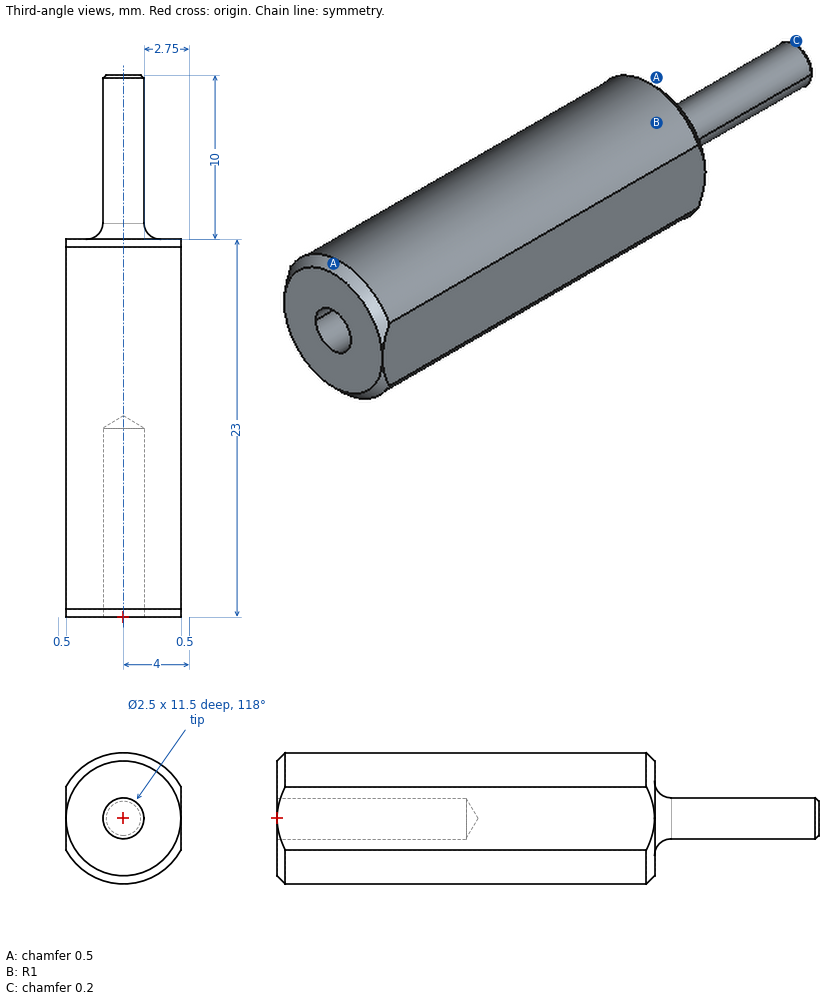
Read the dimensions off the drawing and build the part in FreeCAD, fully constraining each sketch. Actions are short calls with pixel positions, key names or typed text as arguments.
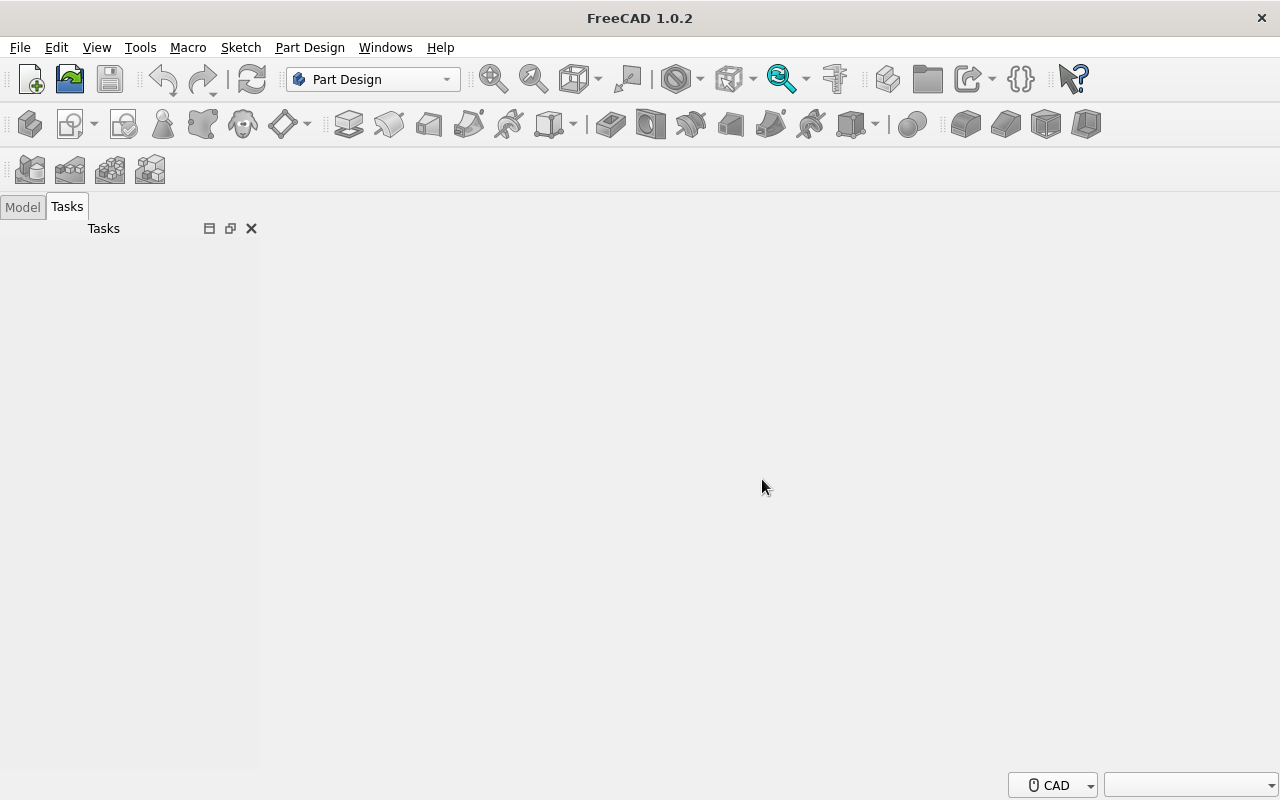
click(30, 80)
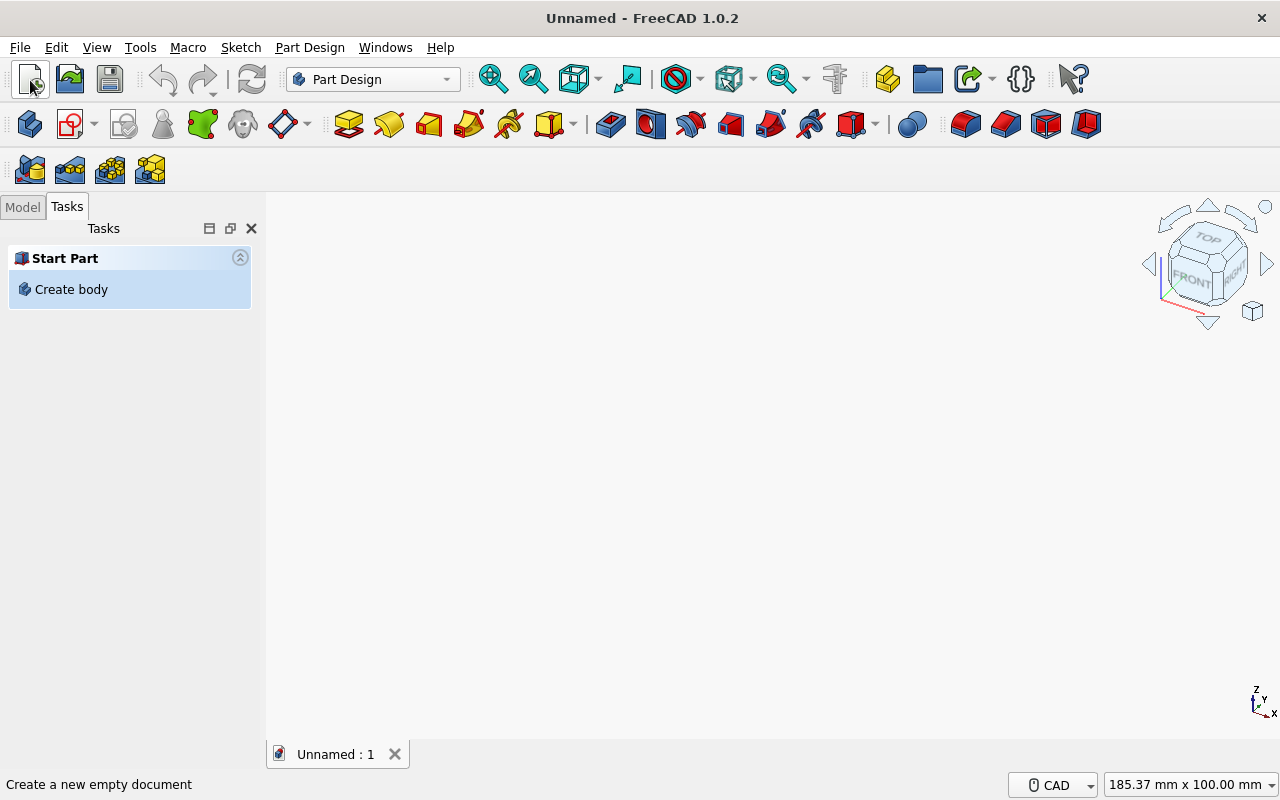
click(70, 124)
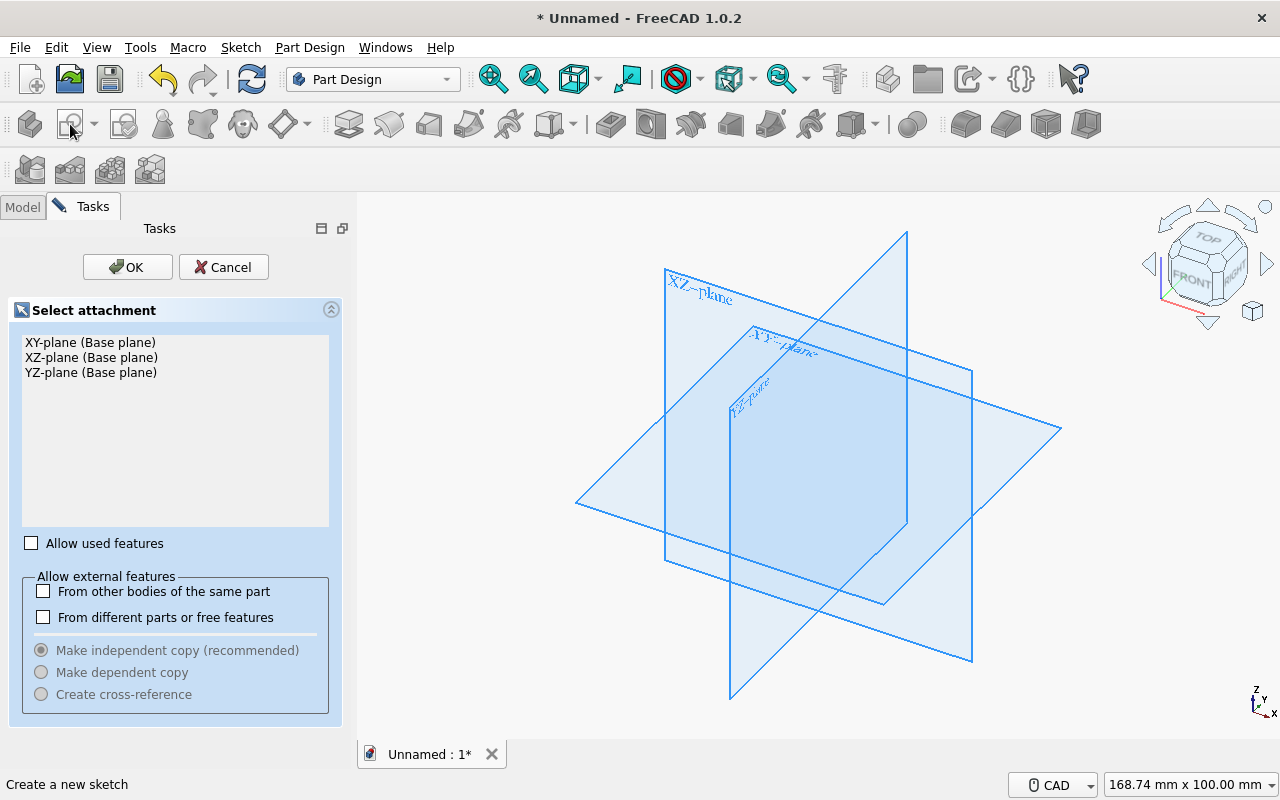
click(82, 342)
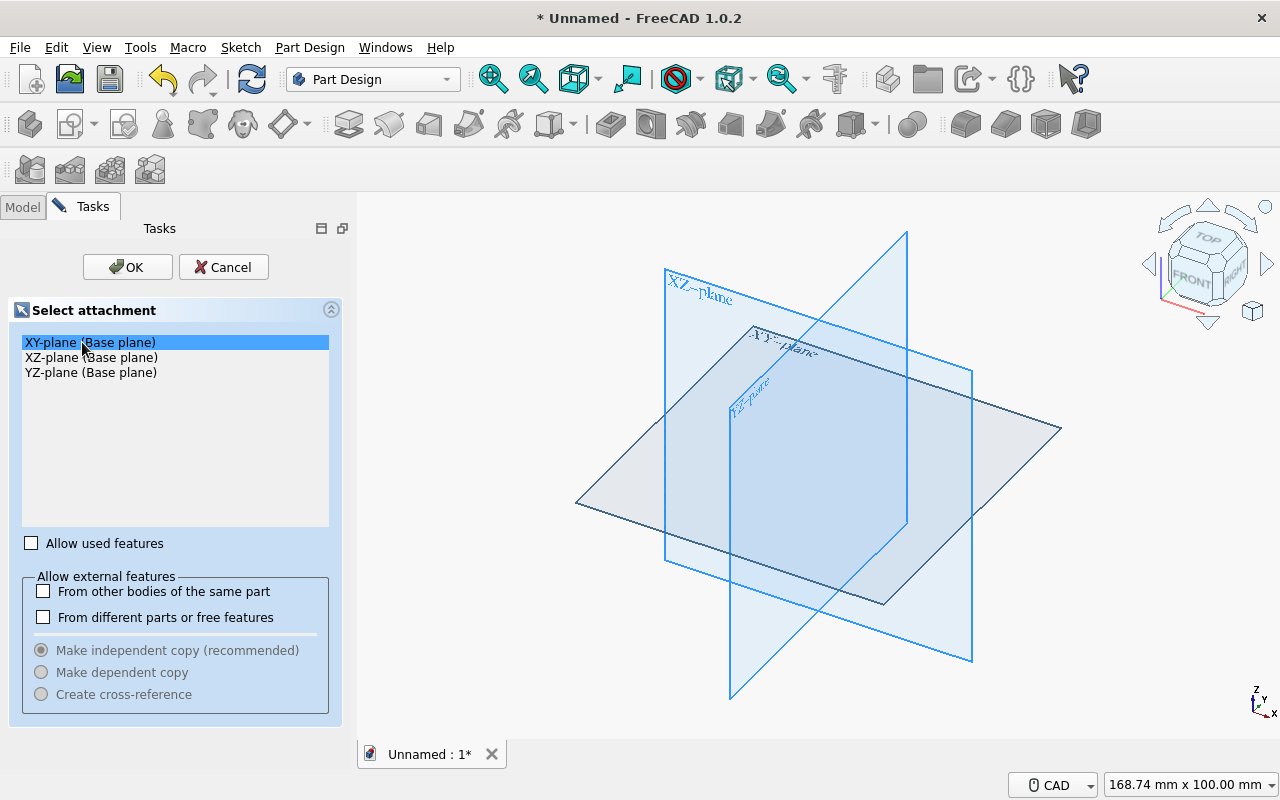
click(128, 267)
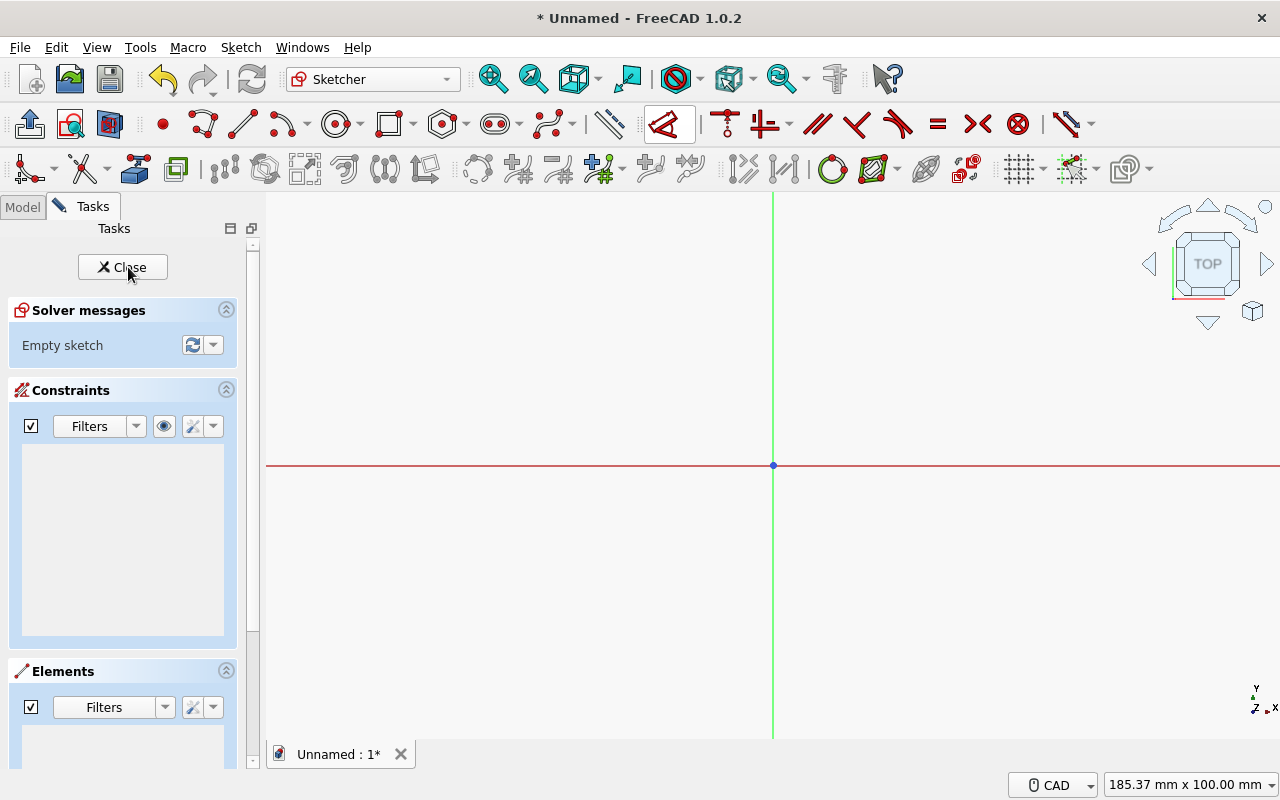
scroll(881, 265, up, 3)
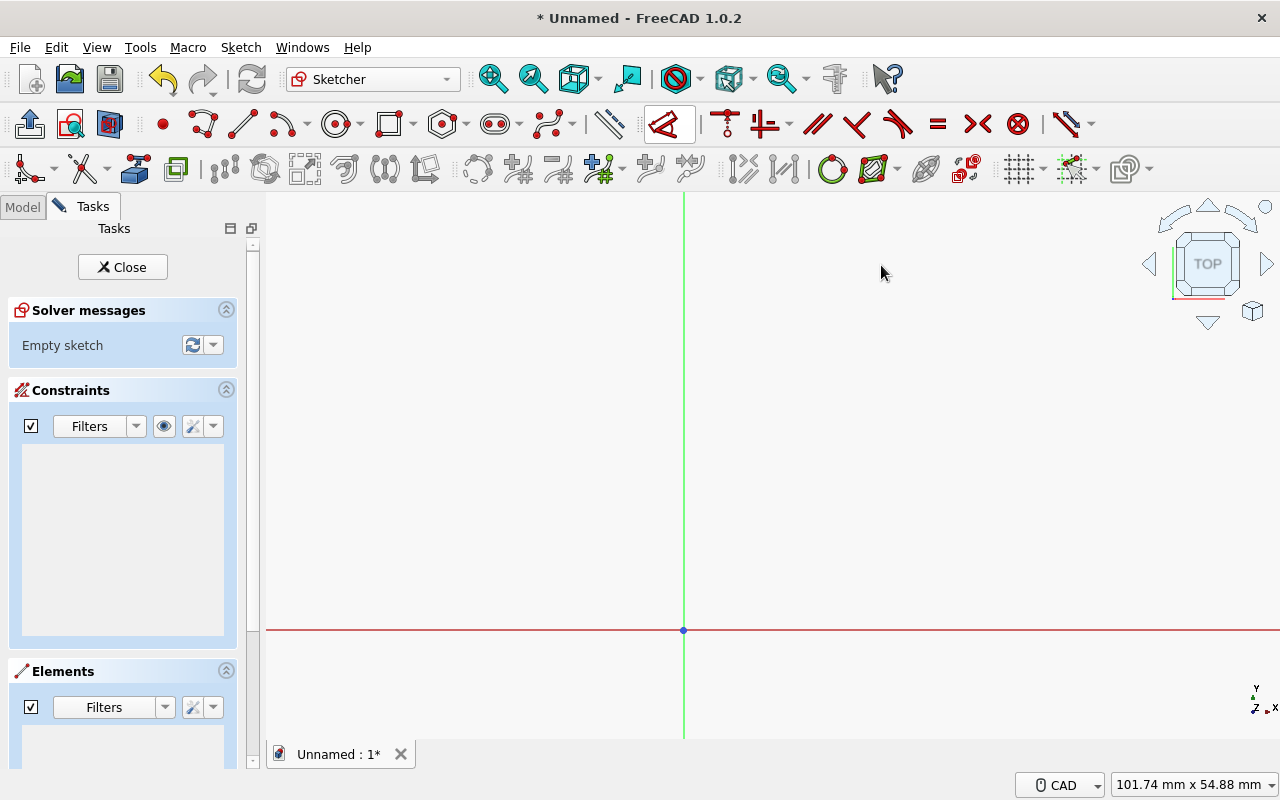
click(204, 124)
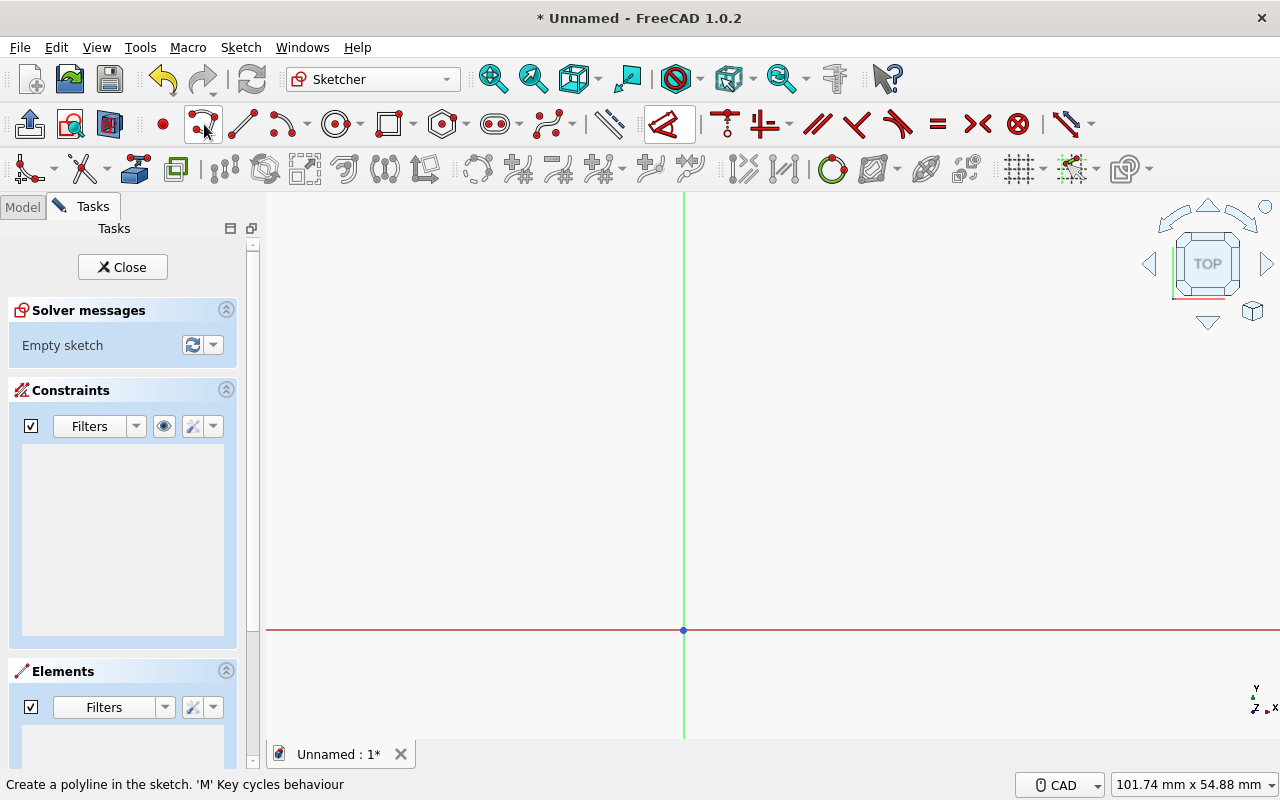
click(684, 630)
click(724, 621)
click(724, 401)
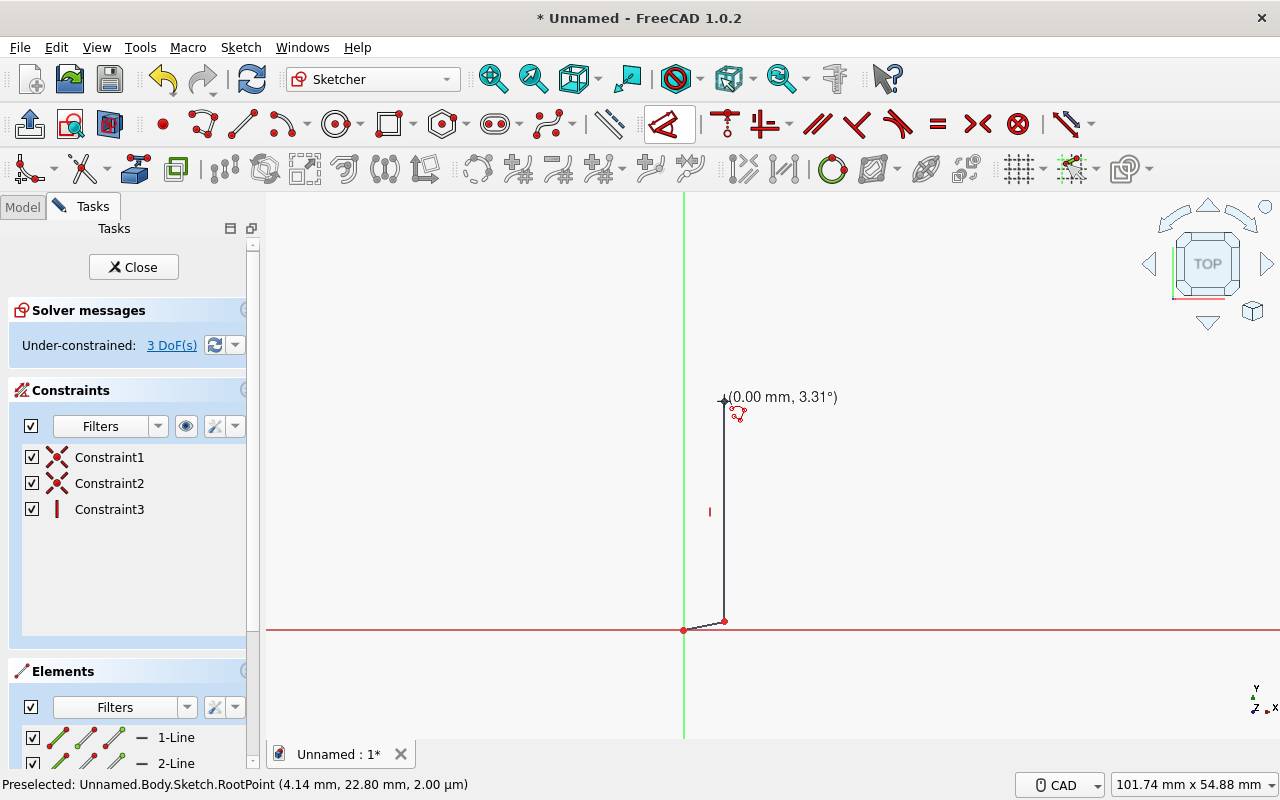
scroll(696, 401, up, 2)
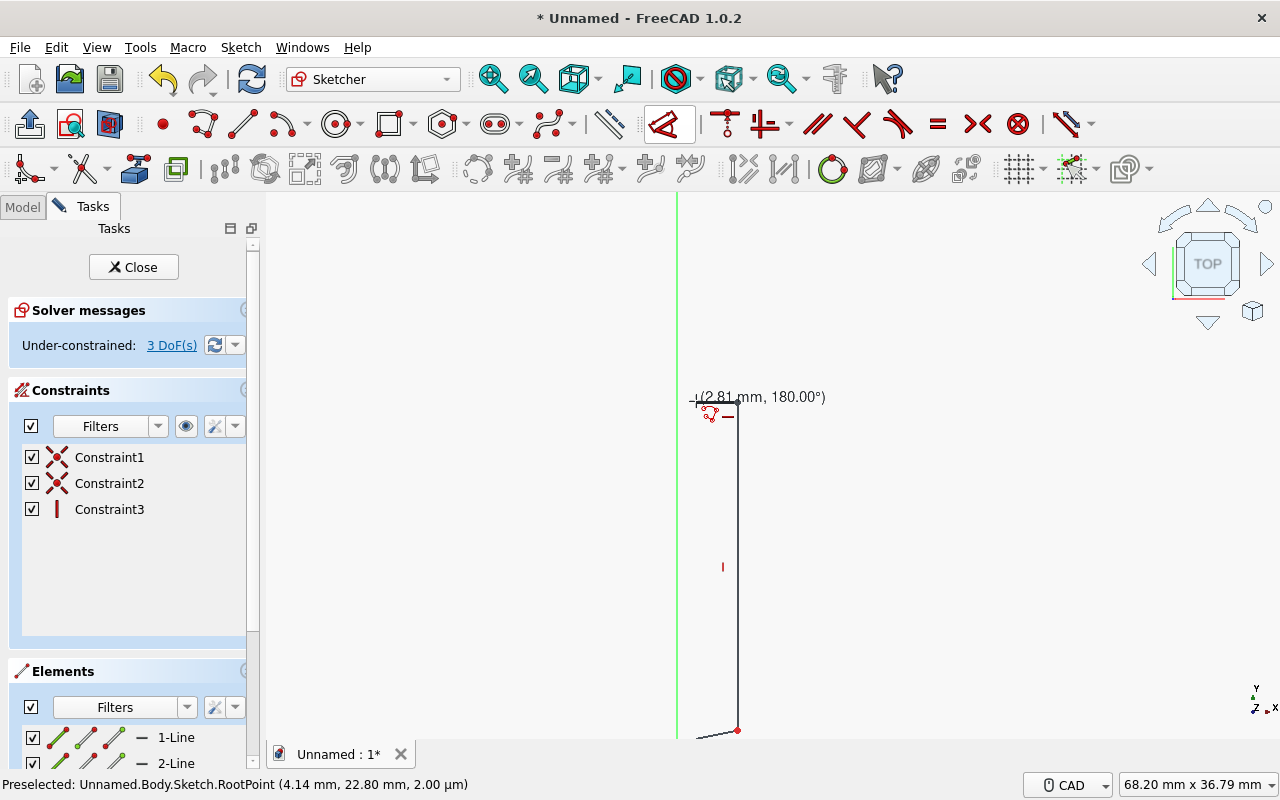
click(696, 401)
click(696, 252)
click(686, 252)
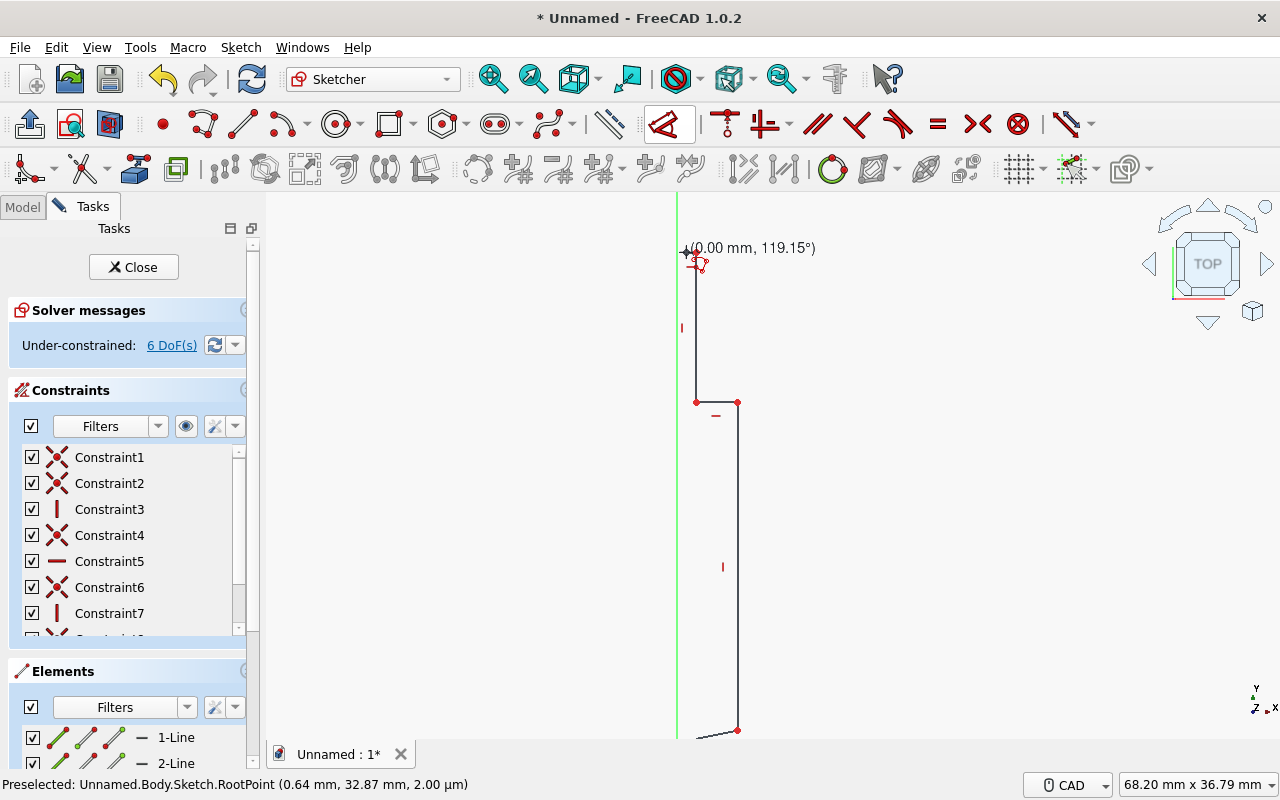
scroll(699, 401, down, 2)